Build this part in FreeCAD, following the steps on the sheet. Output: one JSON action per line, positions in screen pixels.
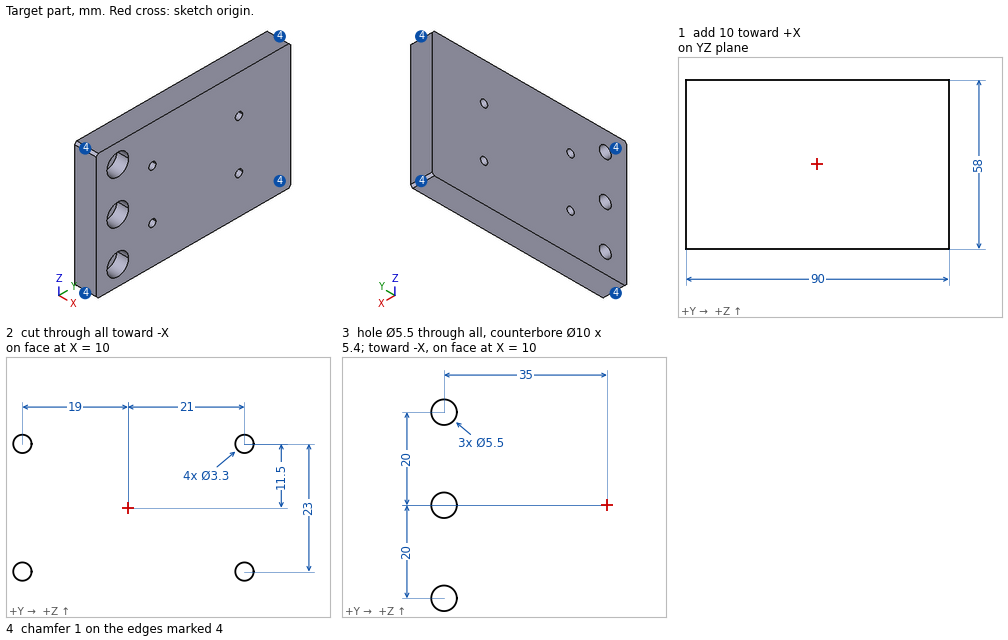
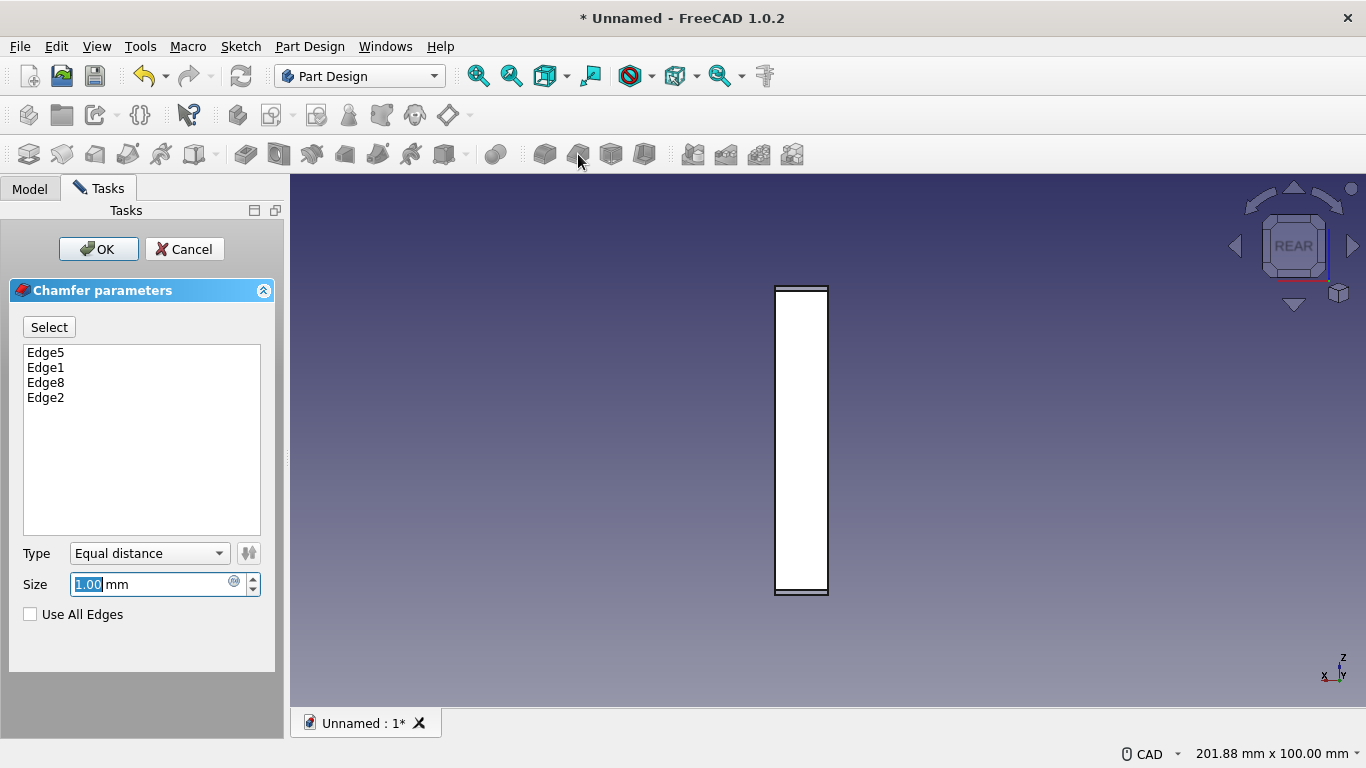
{"action": "type", "text": "1"}
{"action": "key", "text": "Tab"}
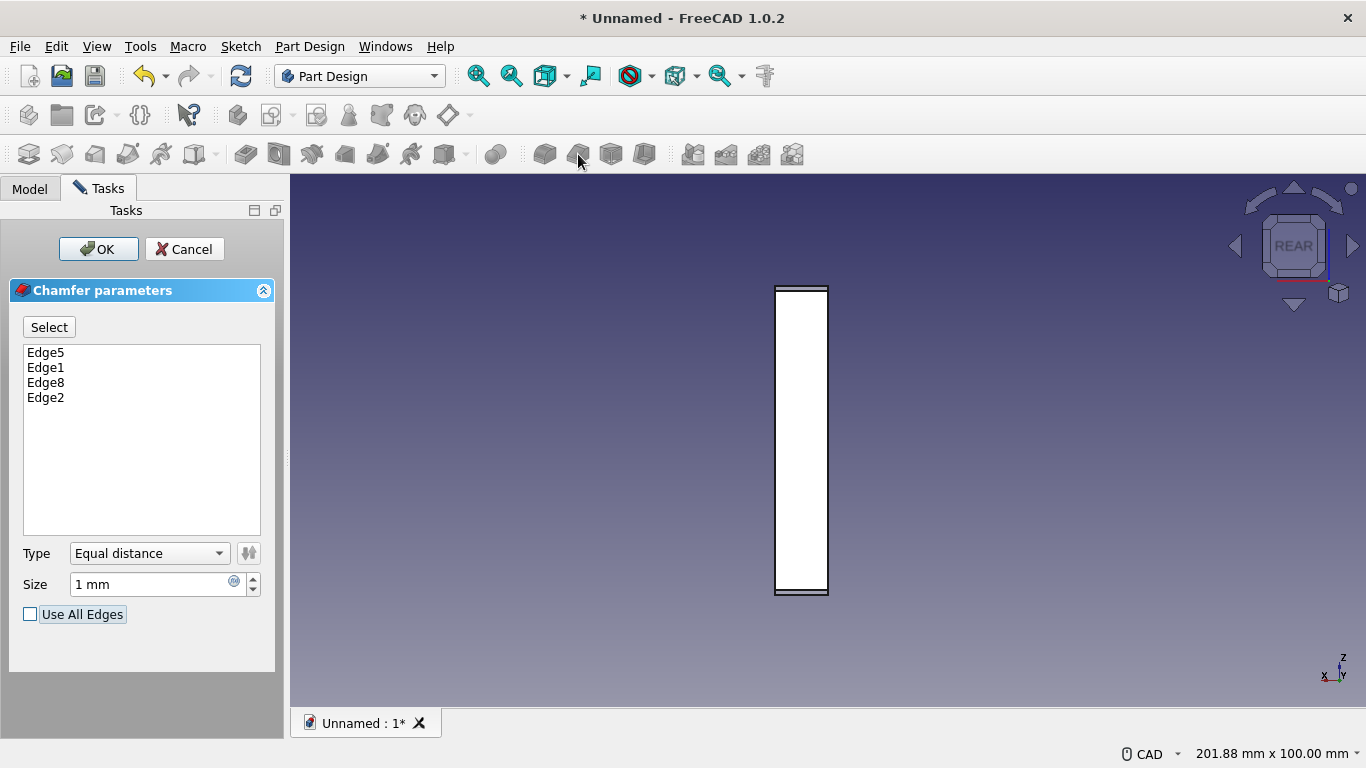
{"action": "left_click", "coordinate": [99, 249]}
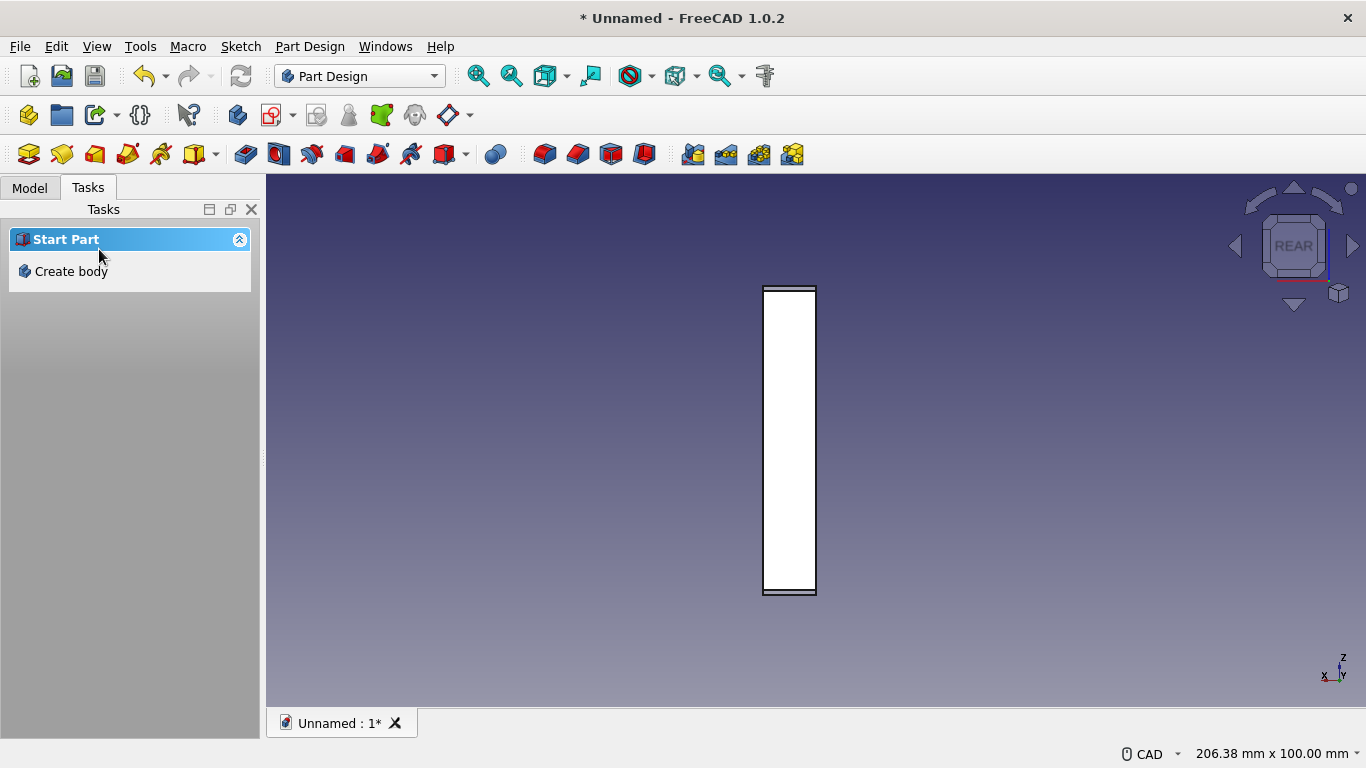
{"action": "key", "text": "0"}